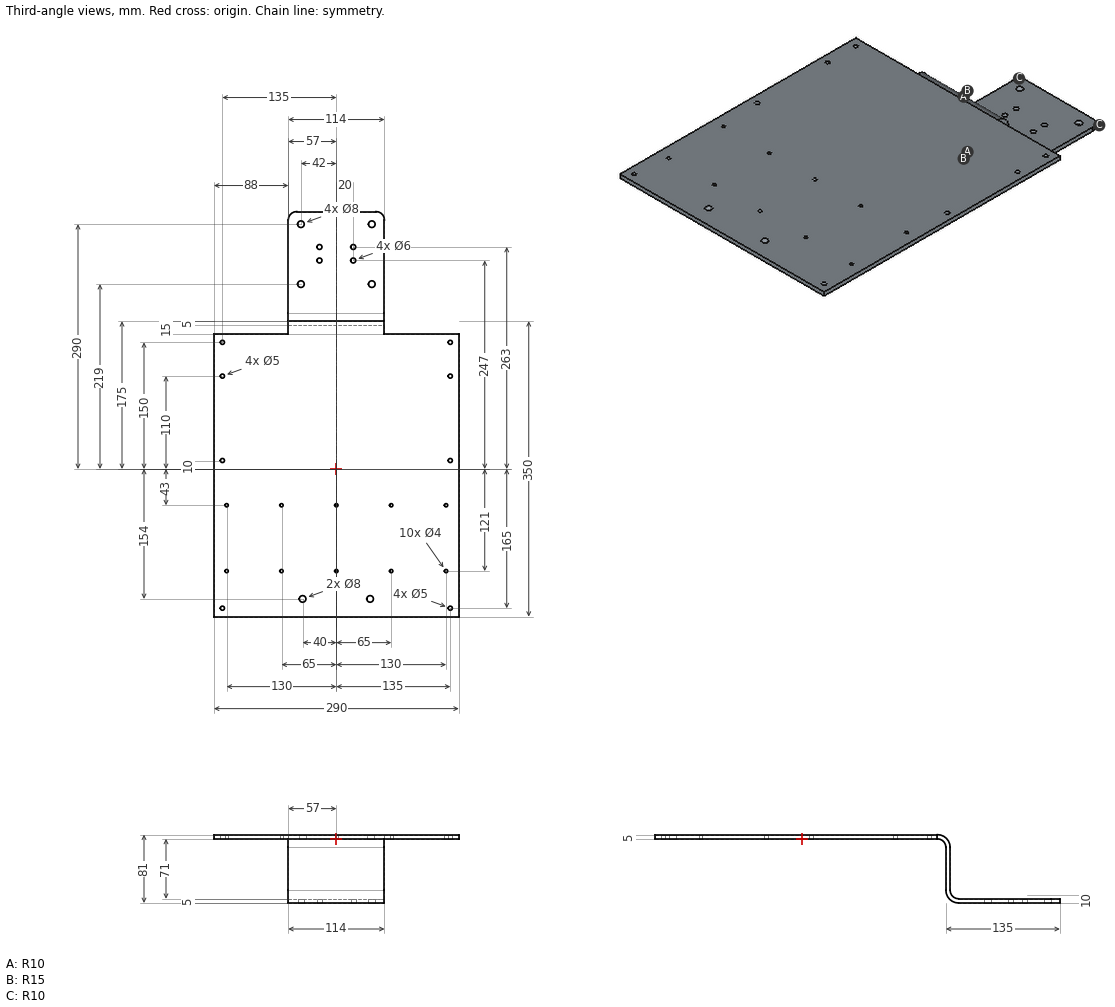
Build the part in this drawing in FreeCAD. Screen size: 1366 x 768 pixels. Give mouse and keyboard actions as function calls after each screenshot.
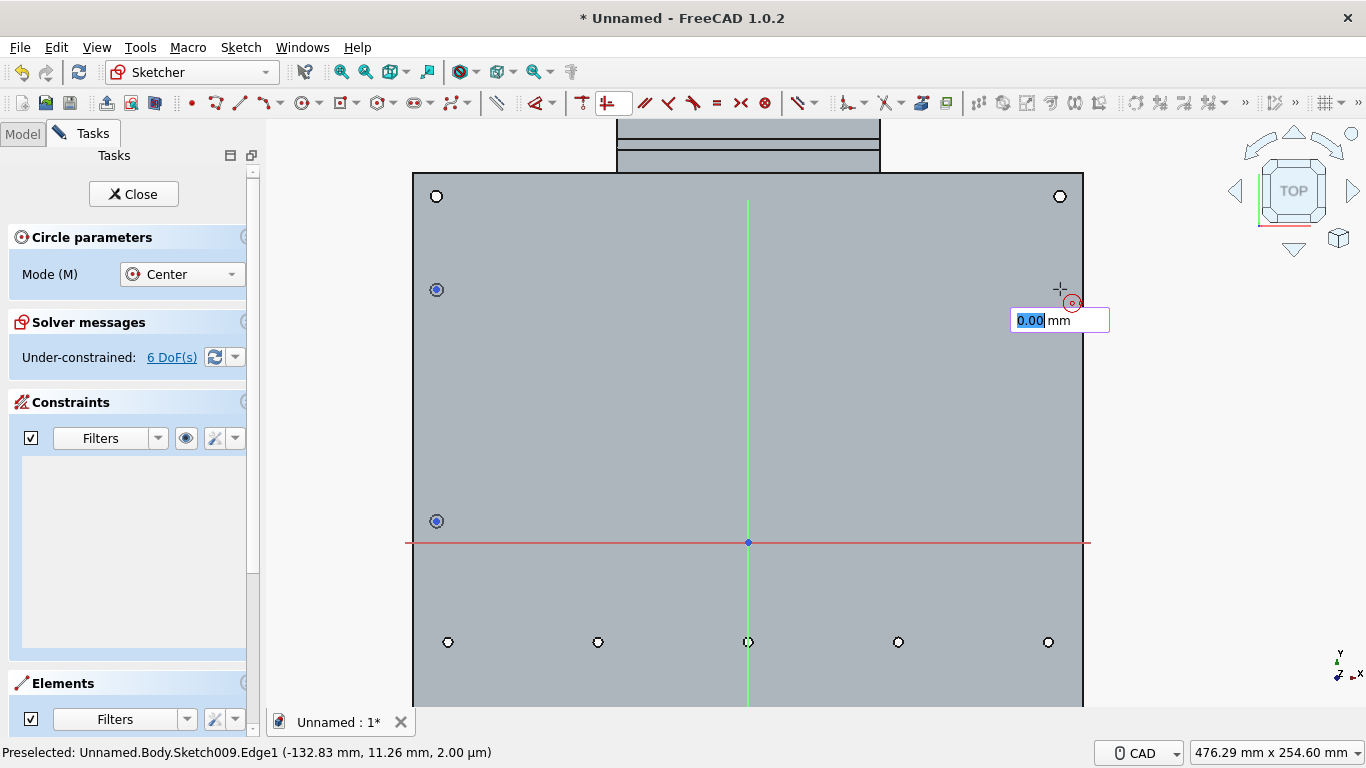
scroll(1064, 285, up, 6)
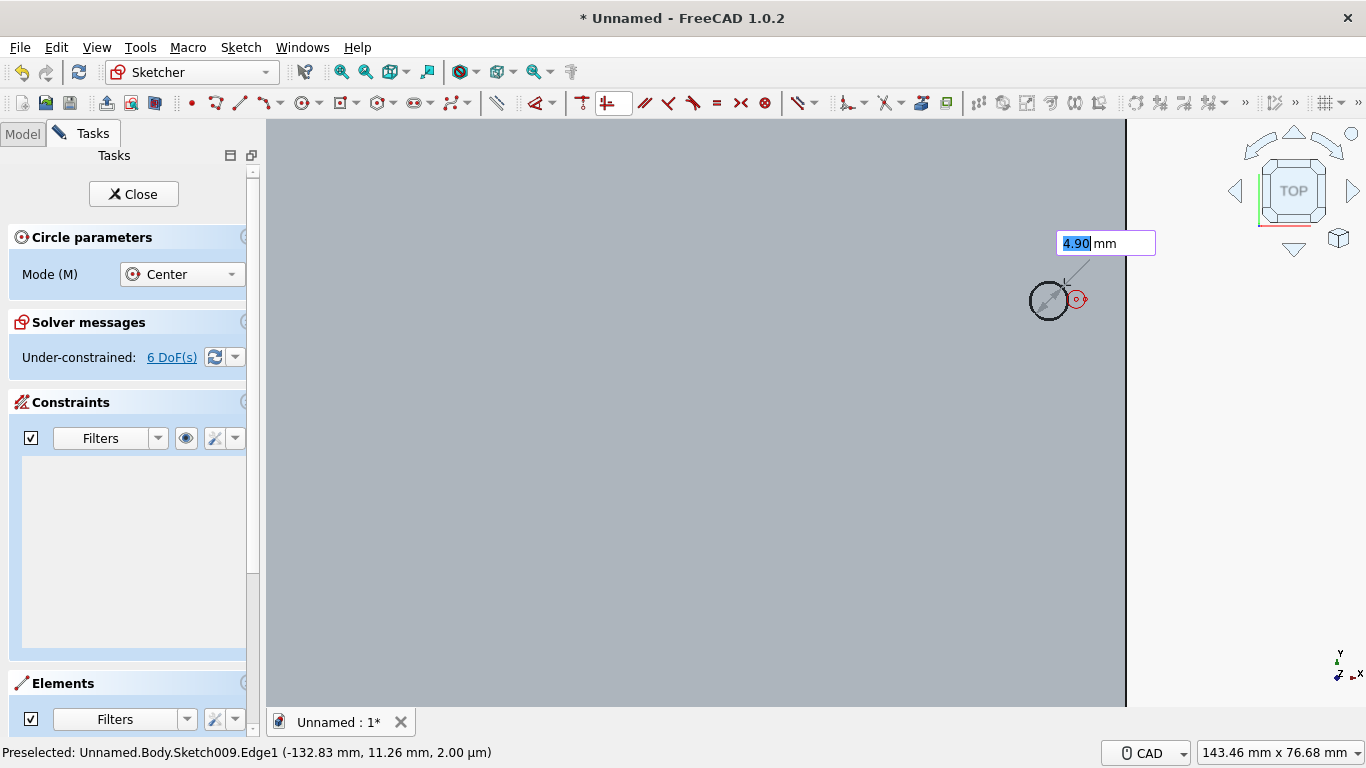
click(1063, 283)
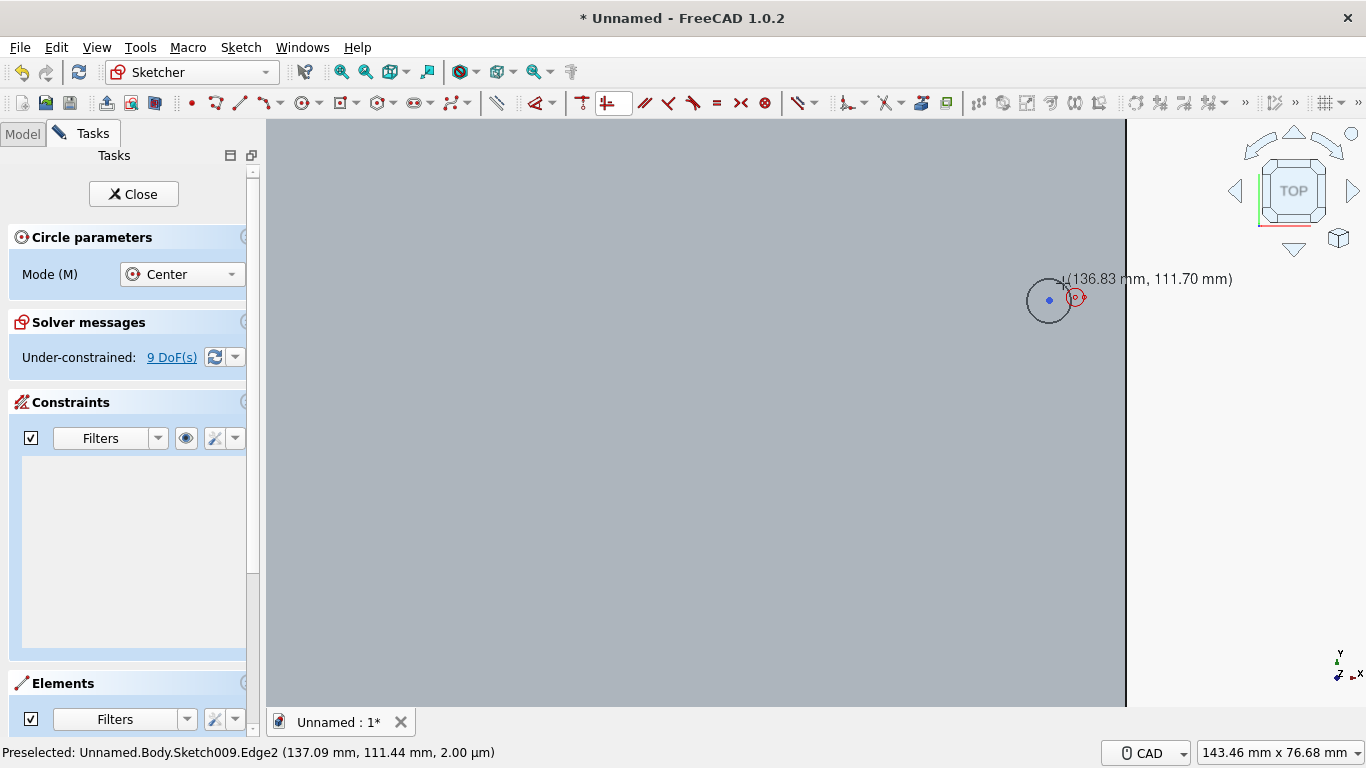
scroll(1064, 285, down, 6)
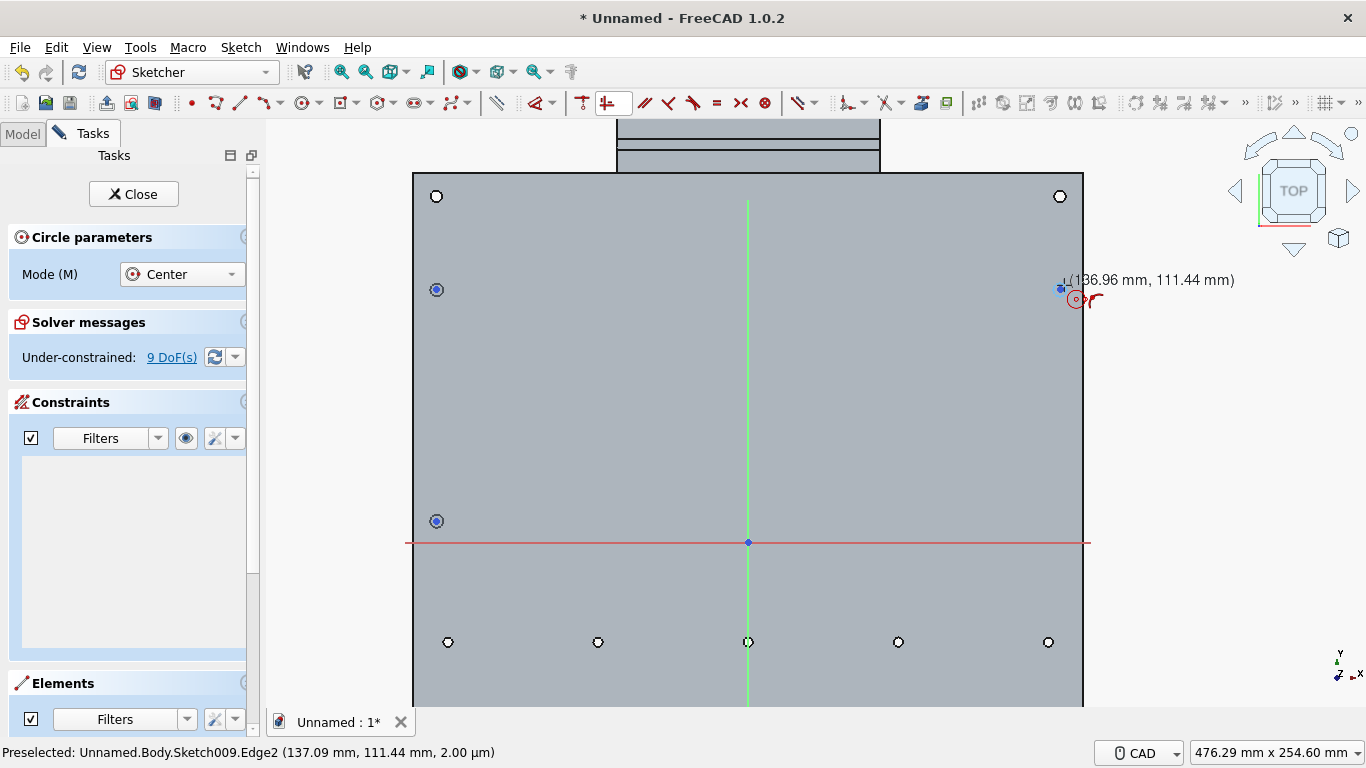
scroll(1060, 520, up, 7)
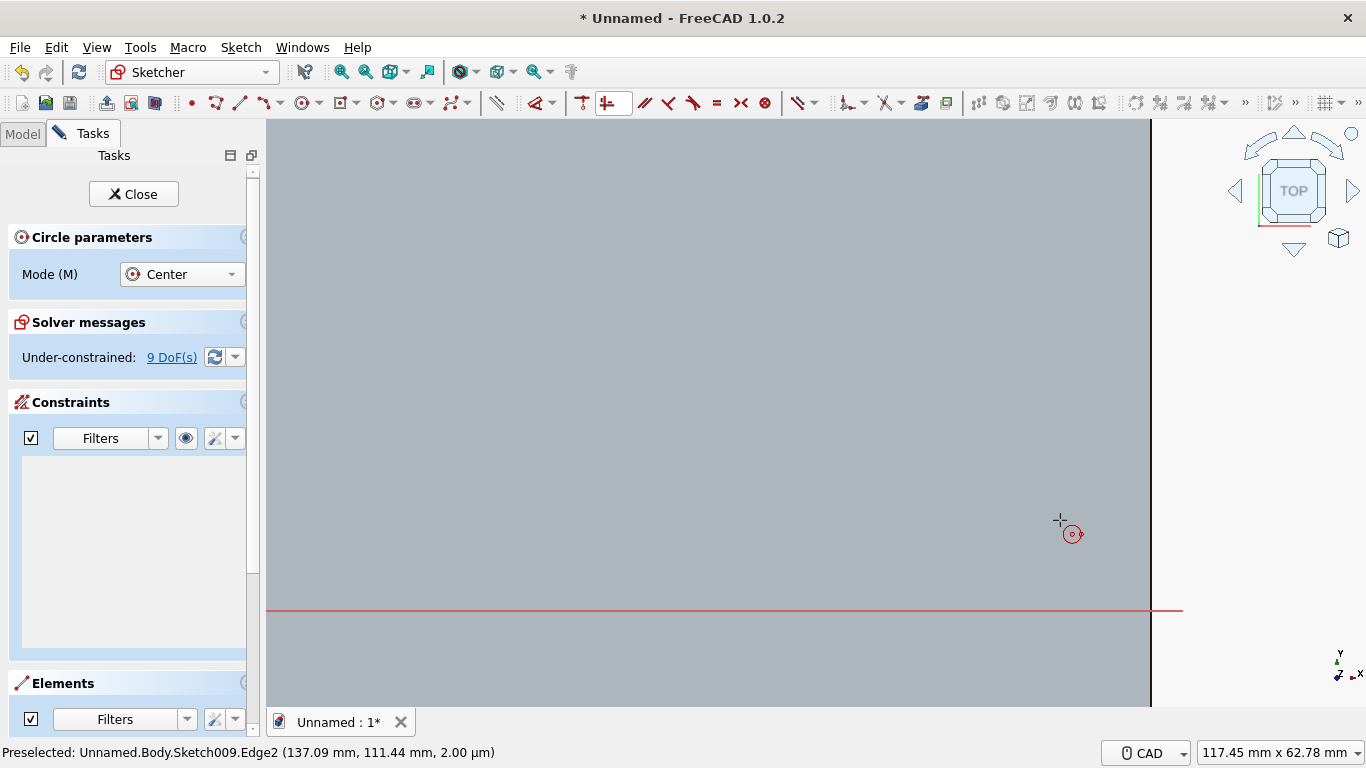
scroll(1060, 521, down, 7)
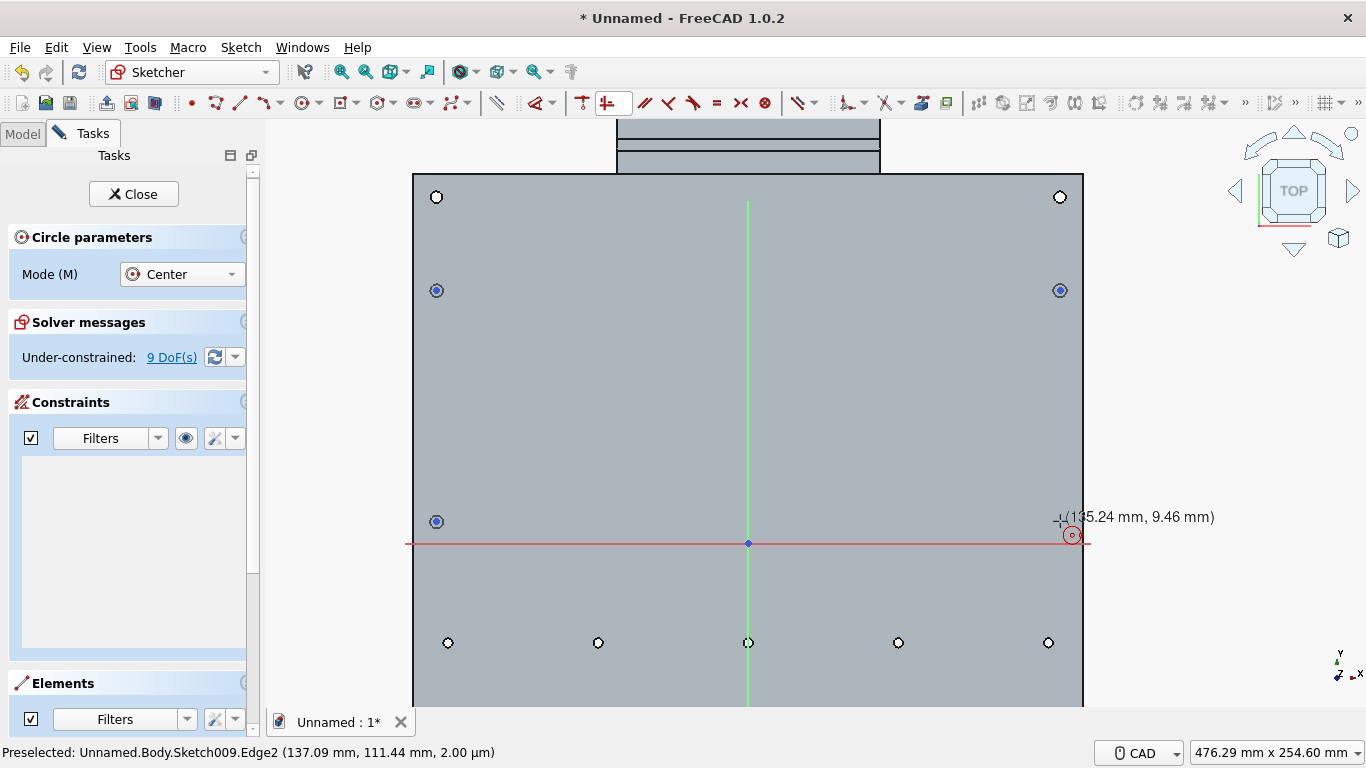
click(1060, 521)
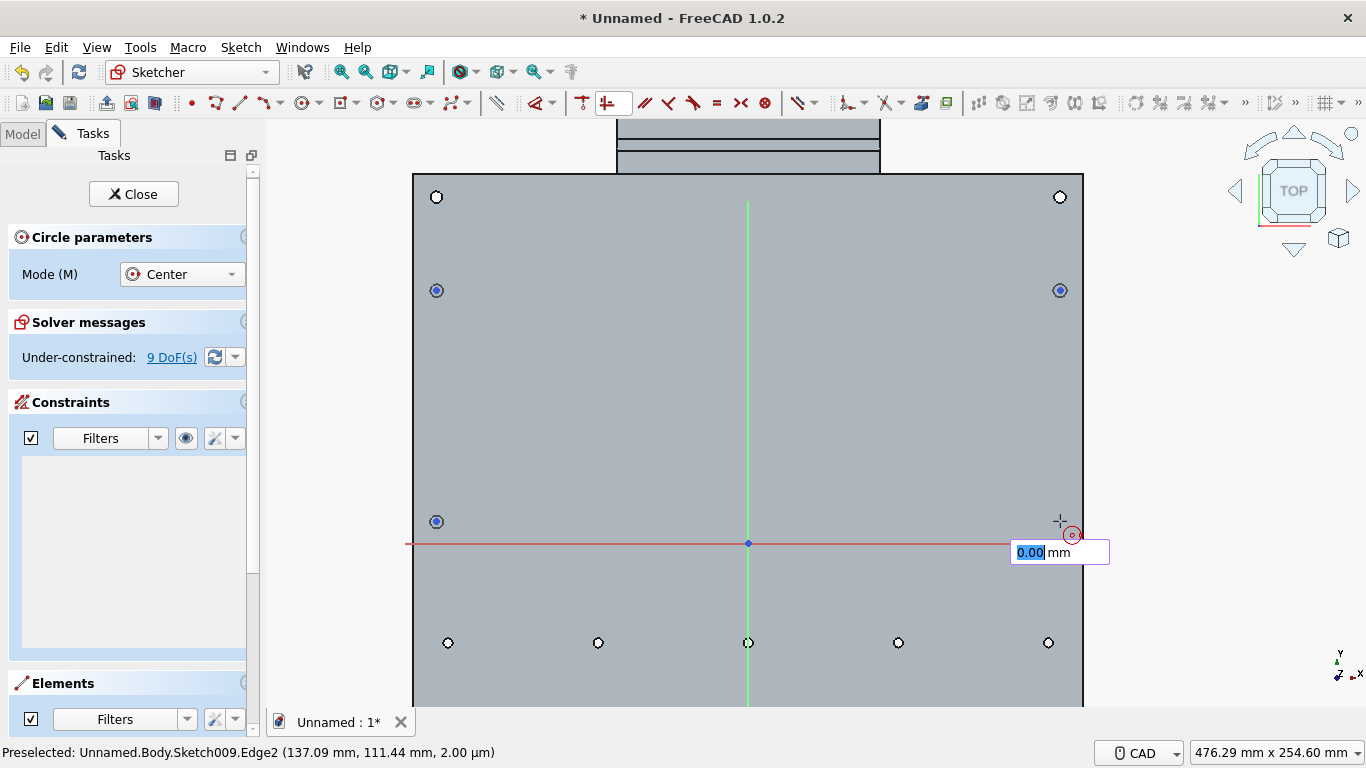
scroll(1064, 516, up, 6)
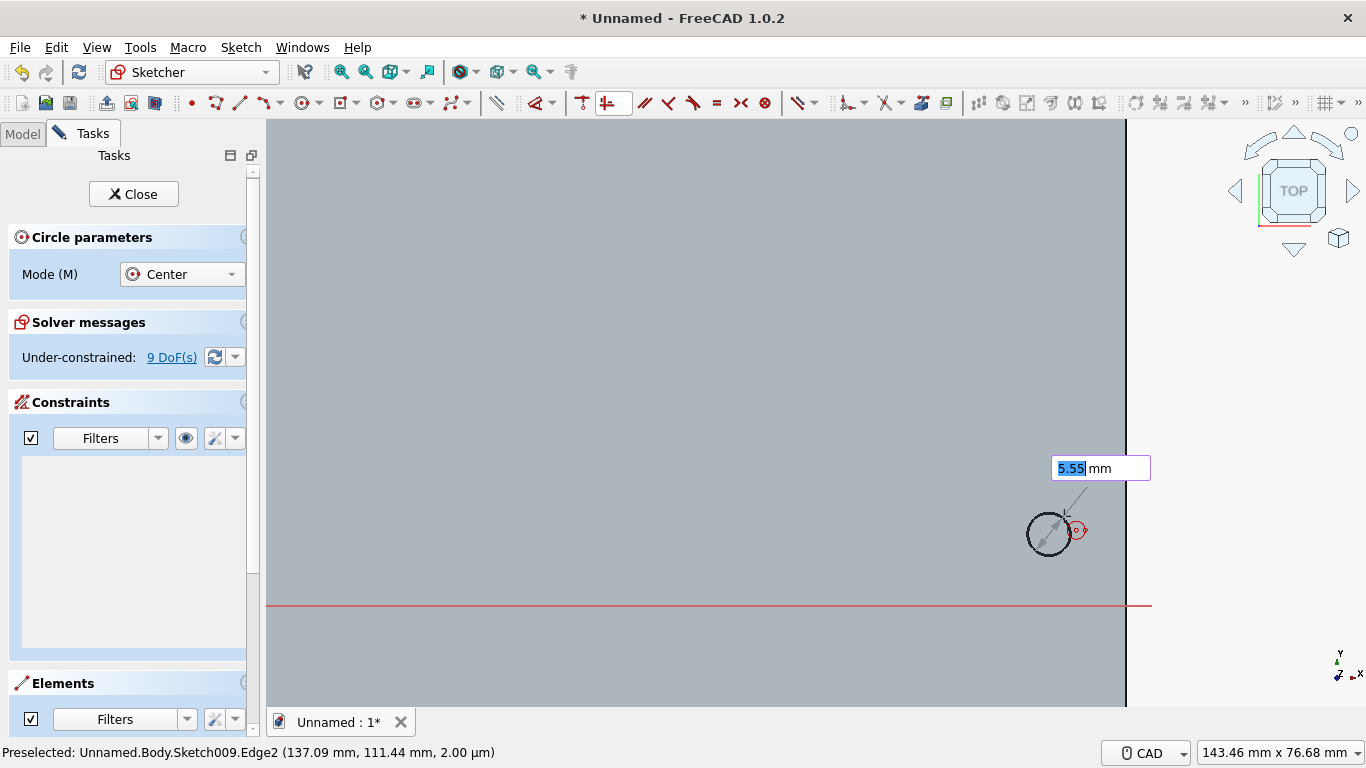
click(1063, 516)
key(Escape)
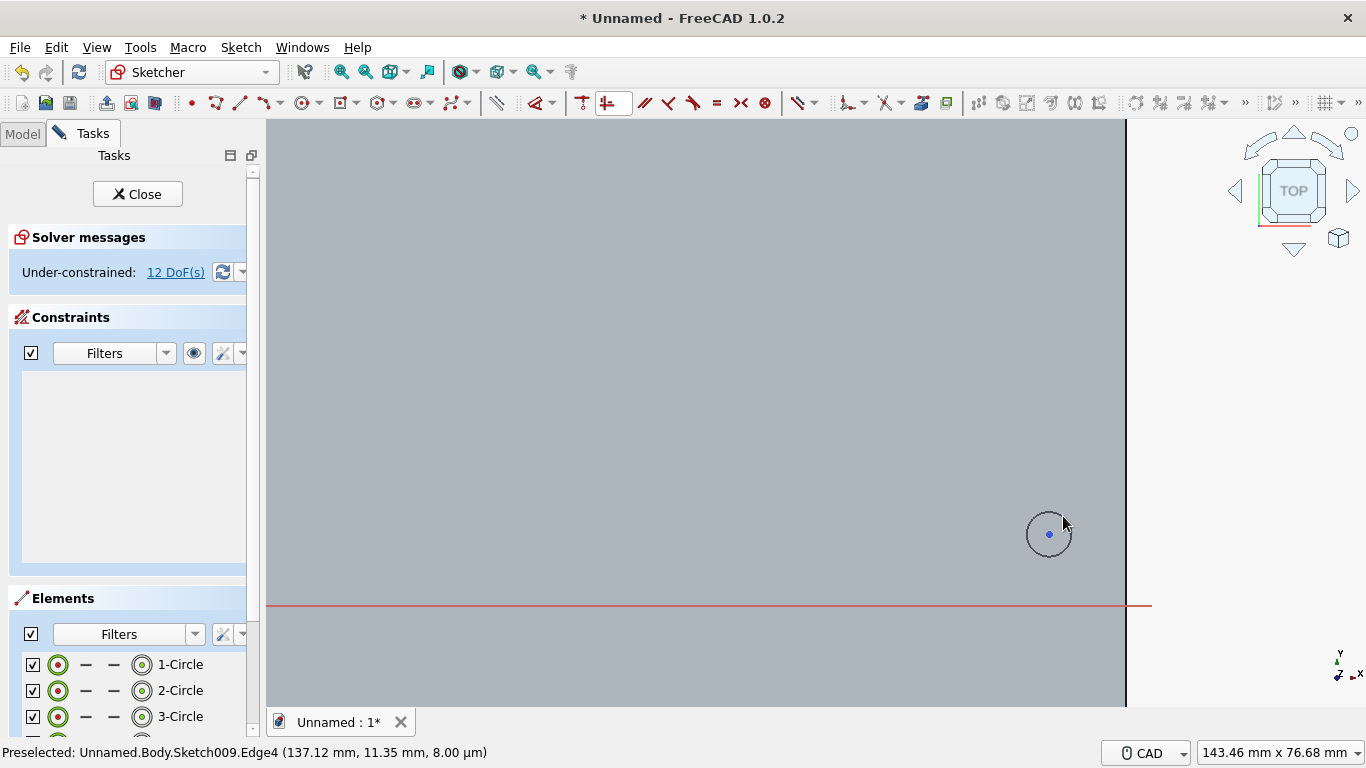
scroll(1064, 516, down, 6)